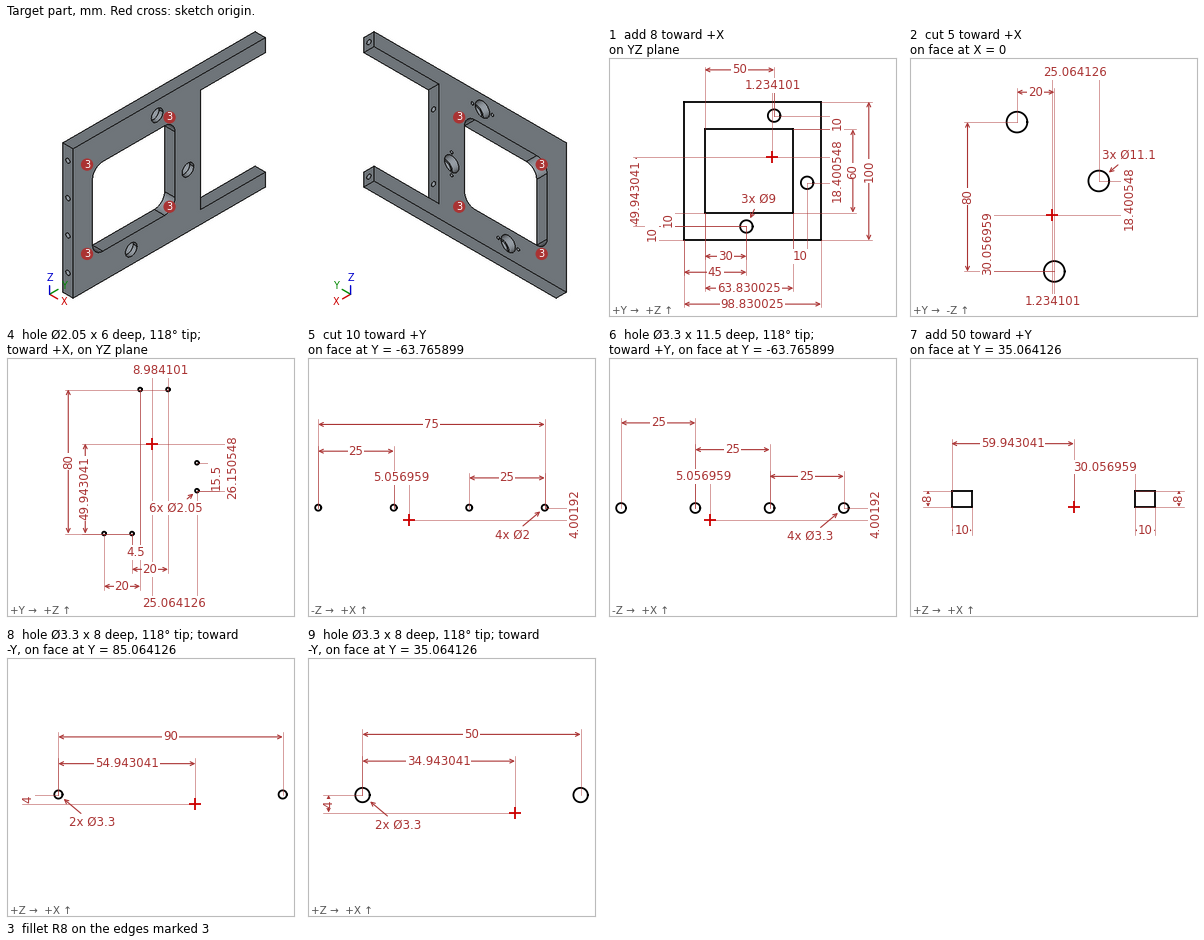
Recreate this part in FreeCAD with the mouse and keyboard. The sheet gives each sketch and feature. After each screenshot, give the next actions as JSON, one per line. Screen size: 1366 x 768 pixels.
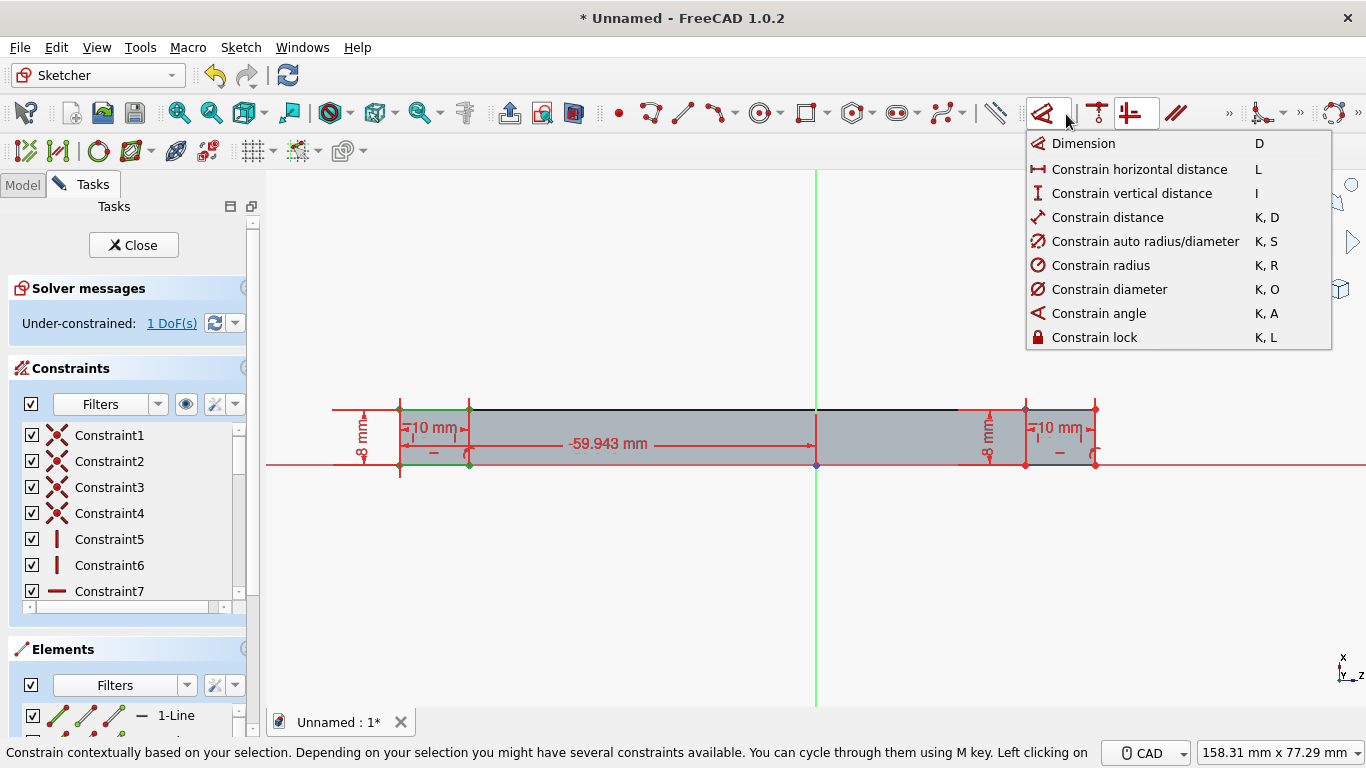
{"action": "left_click", "coordinate": [1179, 169]}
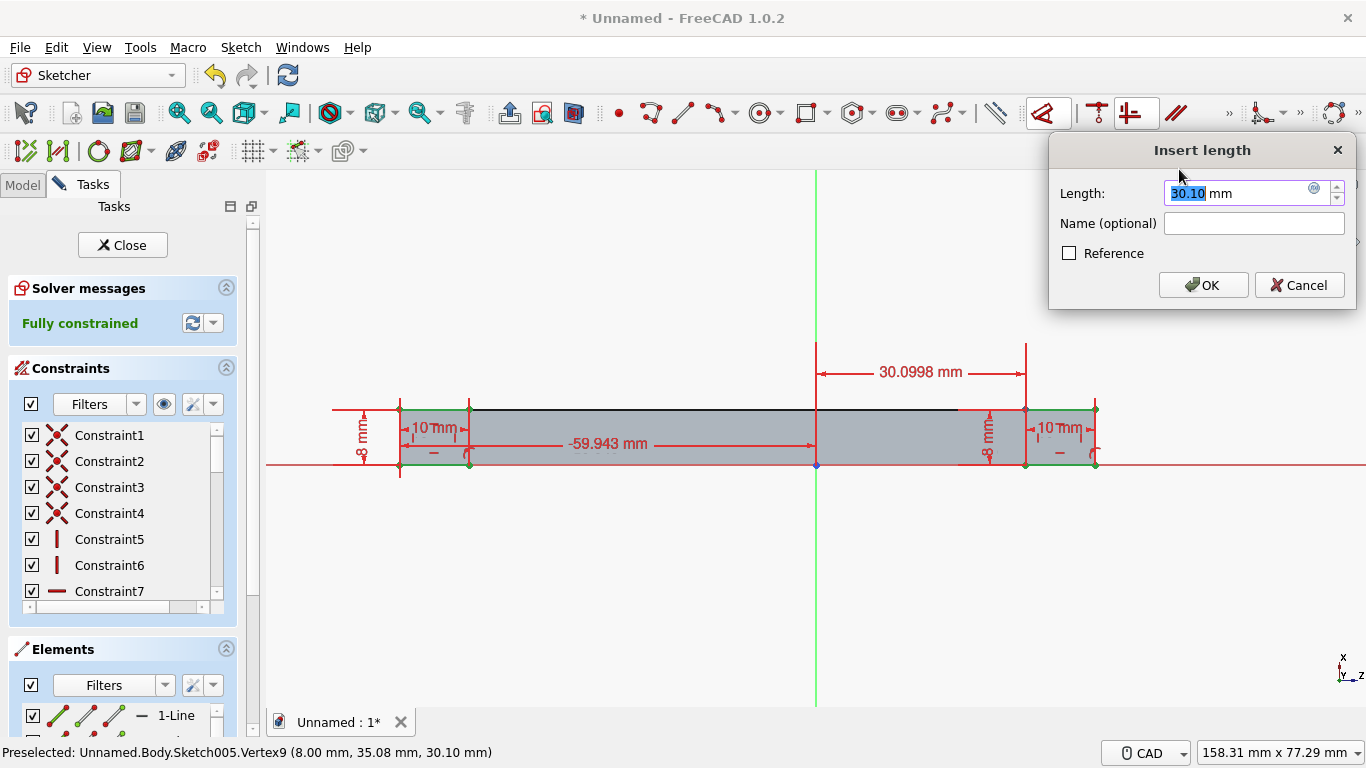
{"action": "type", "text": "30.056959"}
{"action": "key", "text": "Return"}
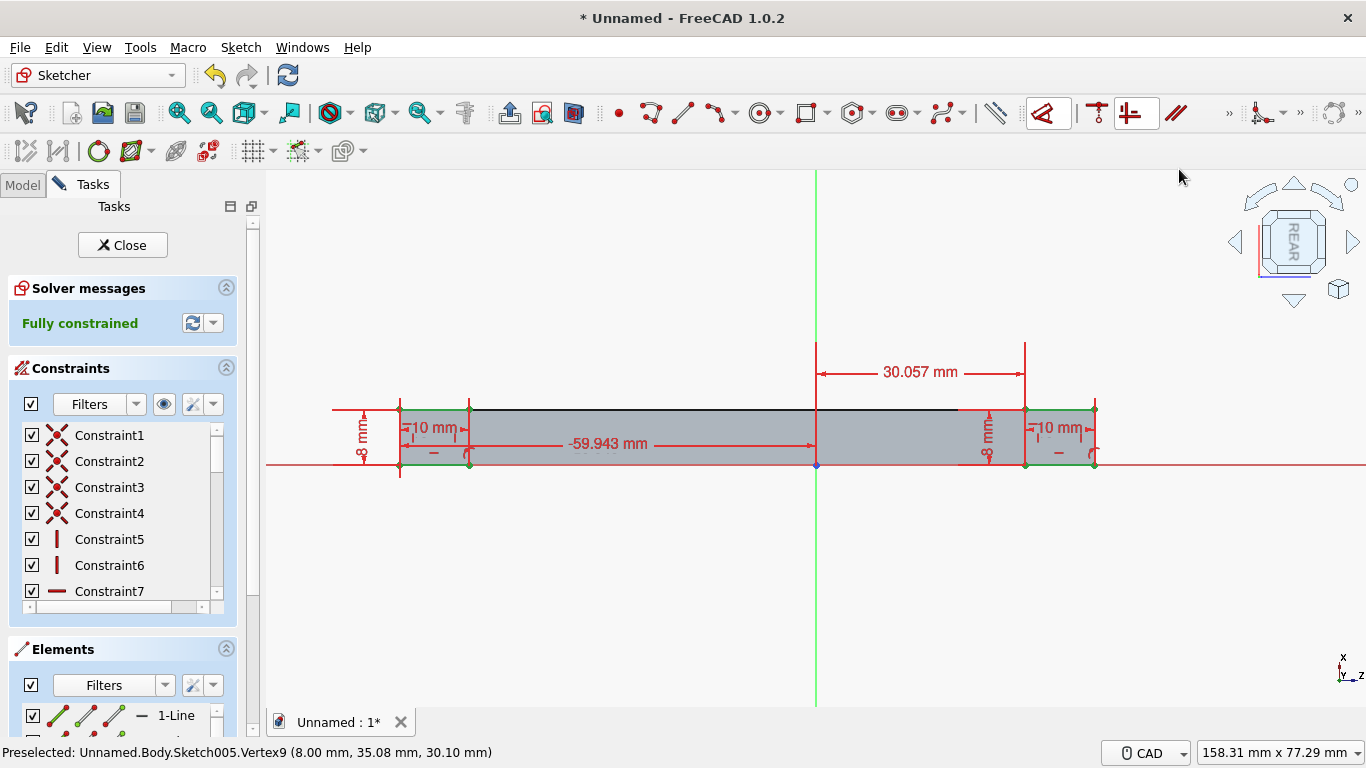
{"action": "left_click", "coordinate": [123, 245]}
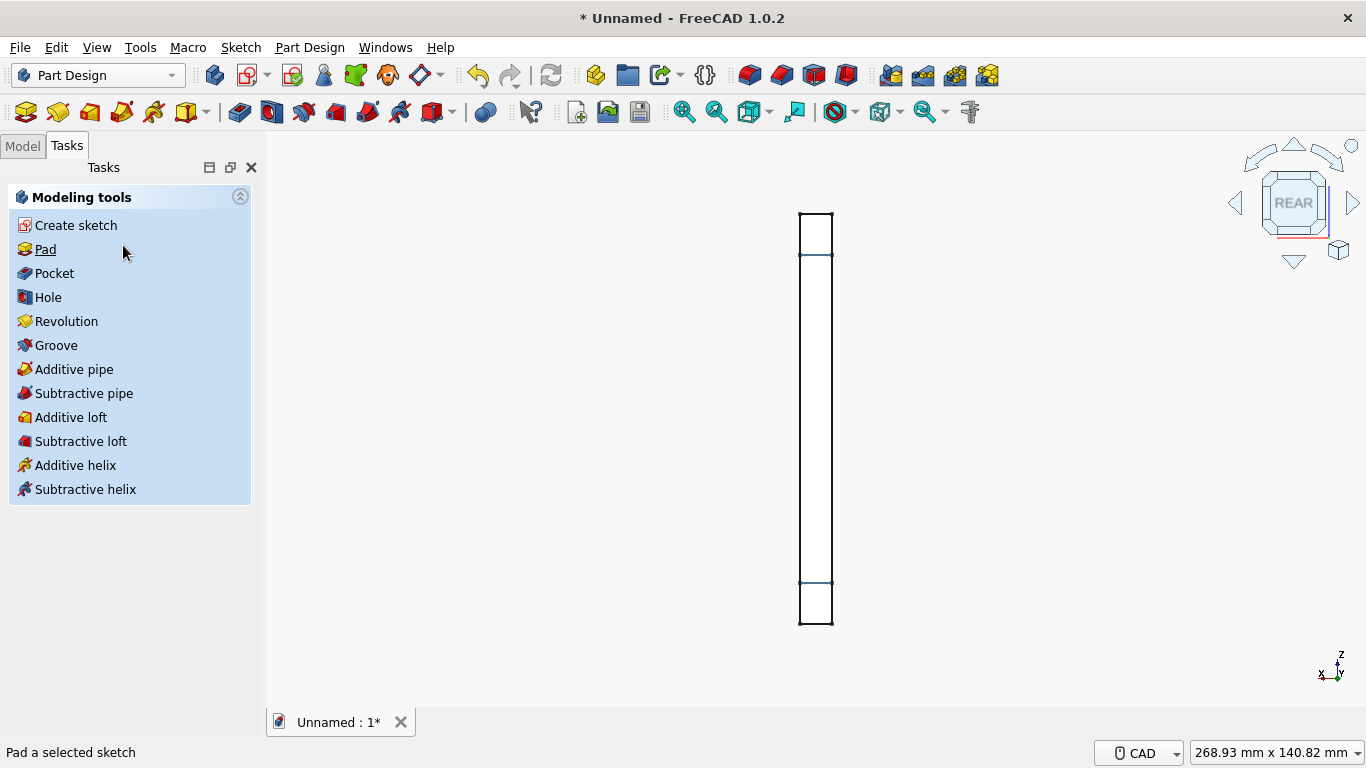
{"action": "left_click", "coordinate": [26, 112]}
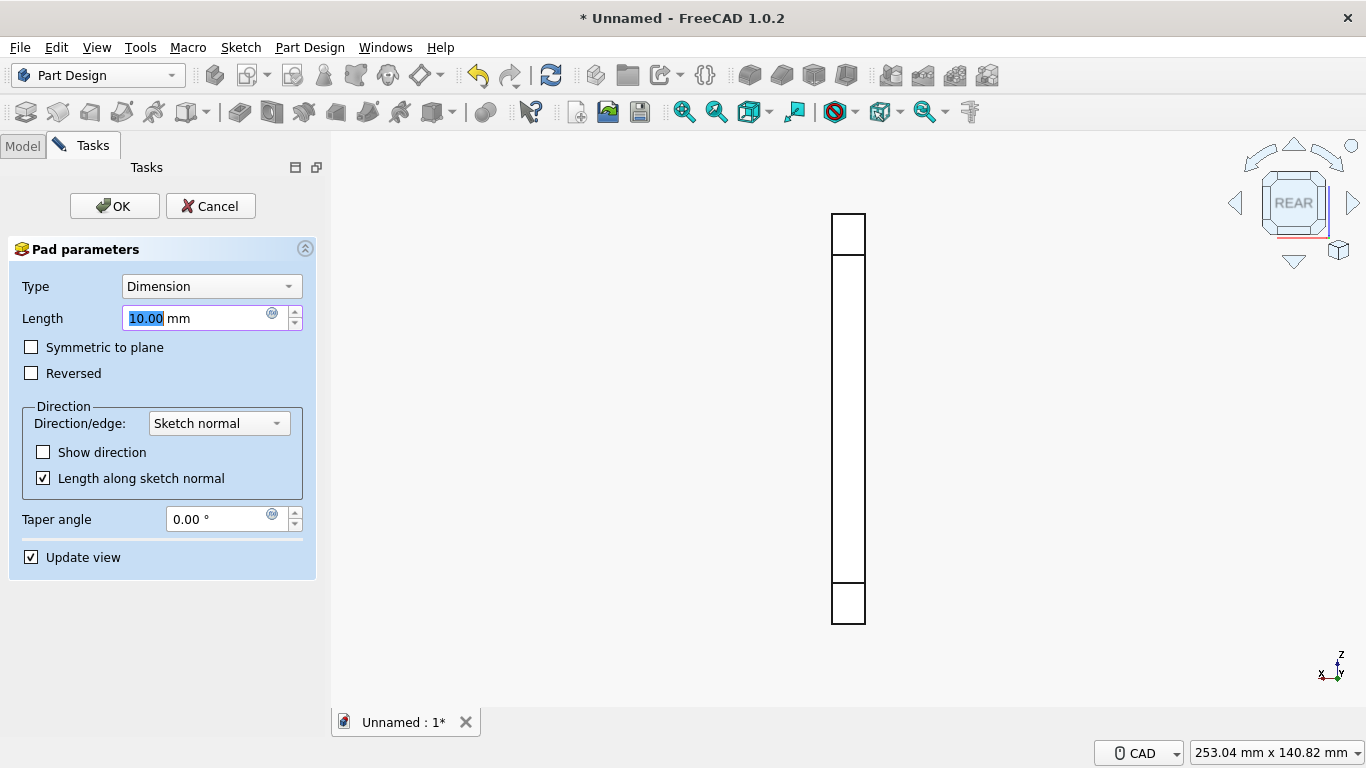
{"action": "type", "text": "50"}
{"action": "key", "text": "Tab"}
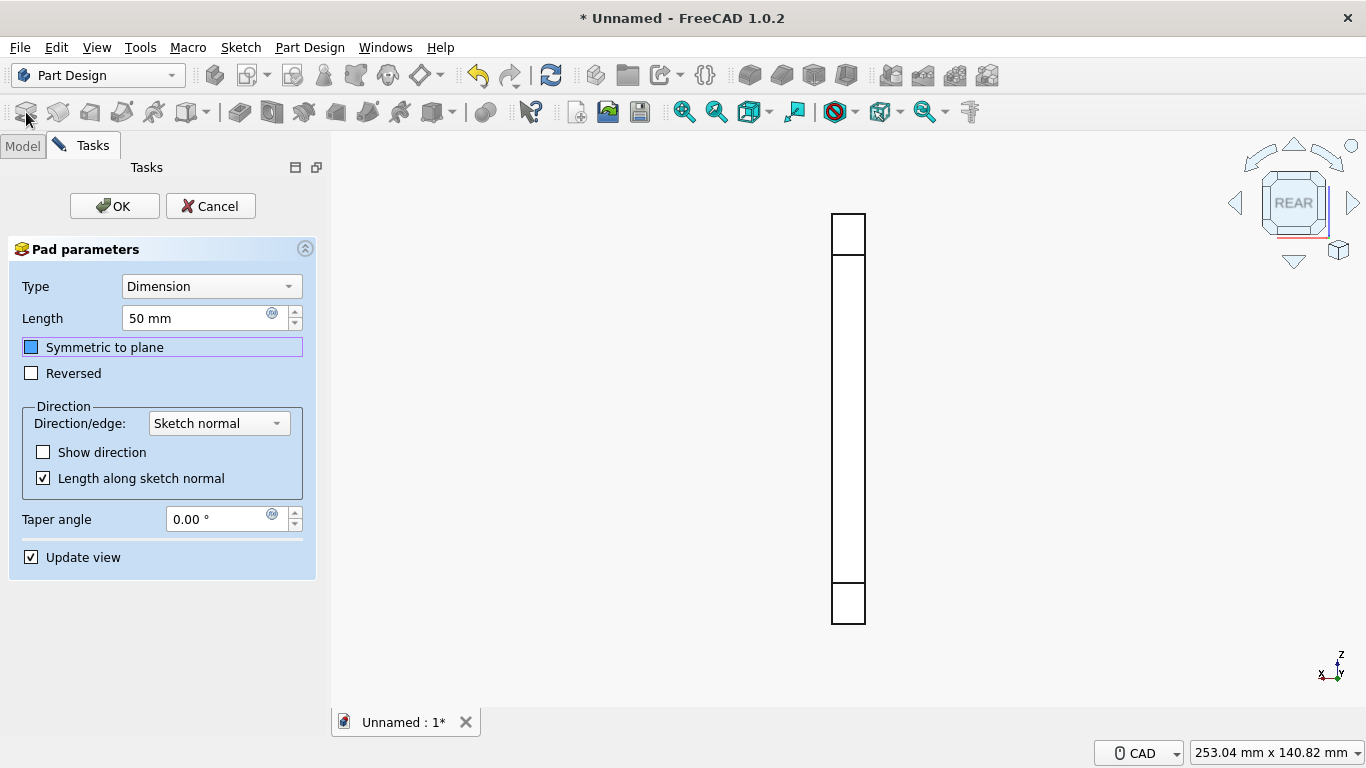
{"action": "left_click", "coordinate": [115, 206]}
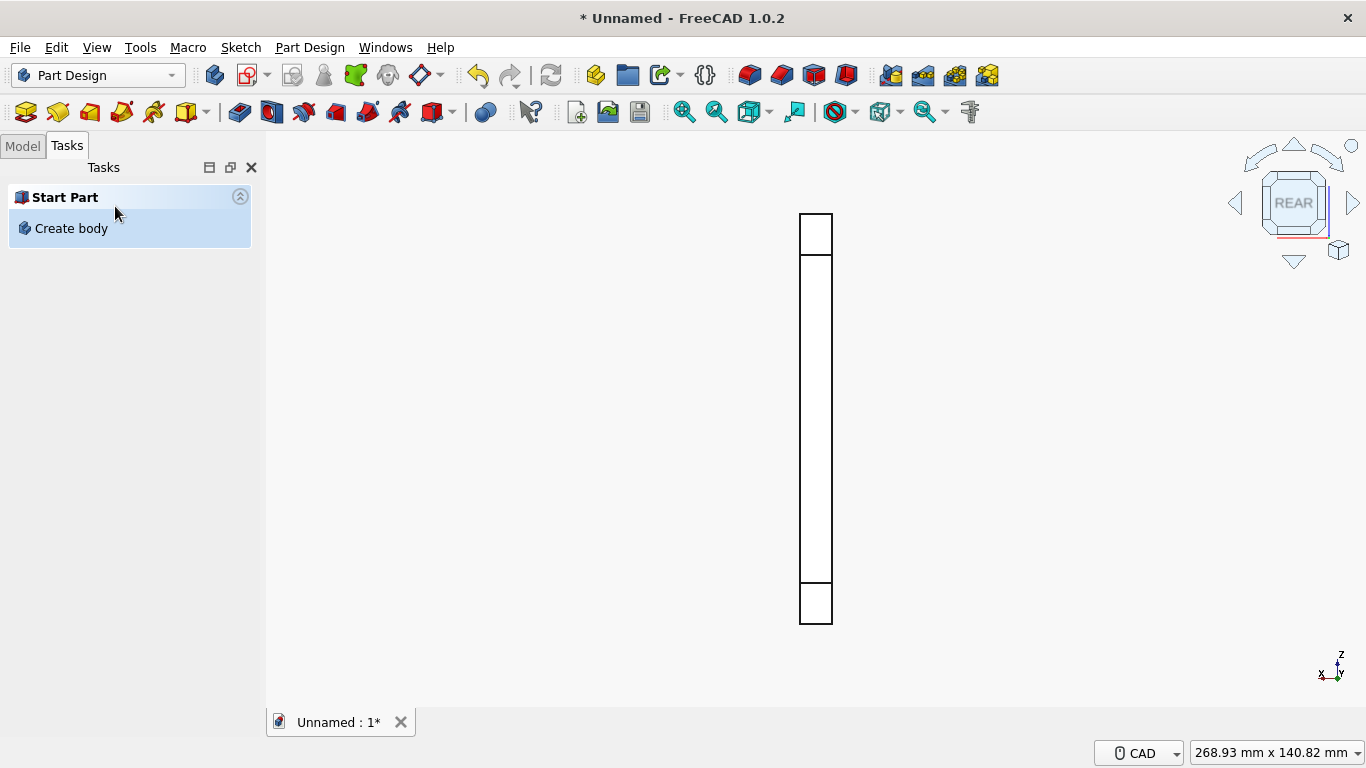
{"action": "left_click", "coordinate": [816, 234]}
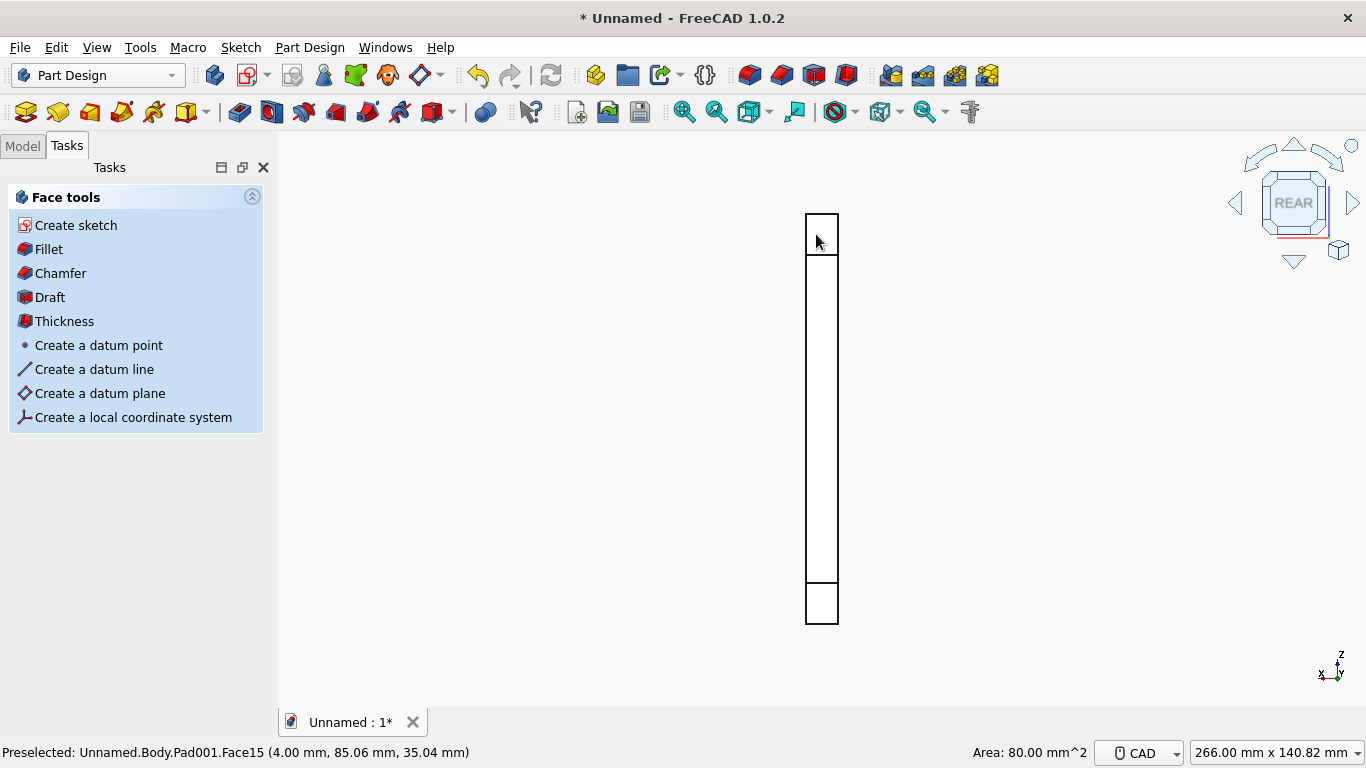
{"action": "left_click", "coordinate": [248, 76]}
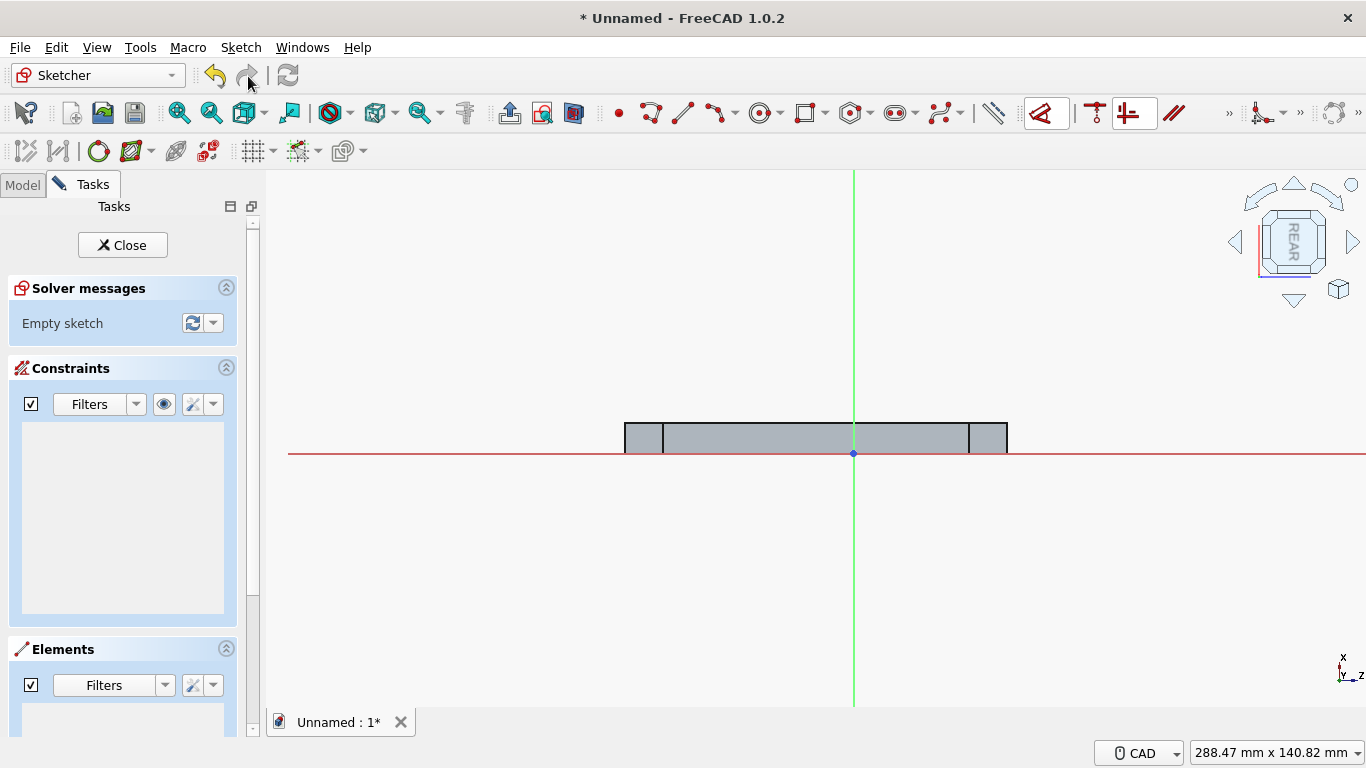
{"action": "scroll", "coordinate": [899, 448], "scroll_direction": "up", "scroll_amount": 3}